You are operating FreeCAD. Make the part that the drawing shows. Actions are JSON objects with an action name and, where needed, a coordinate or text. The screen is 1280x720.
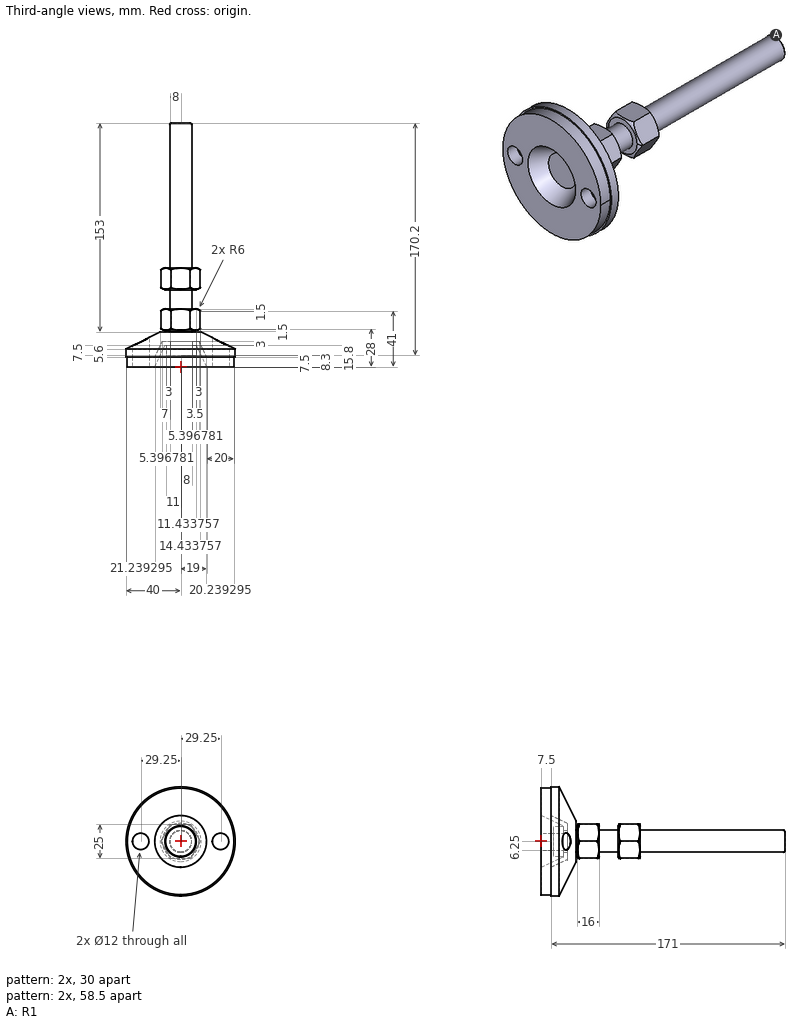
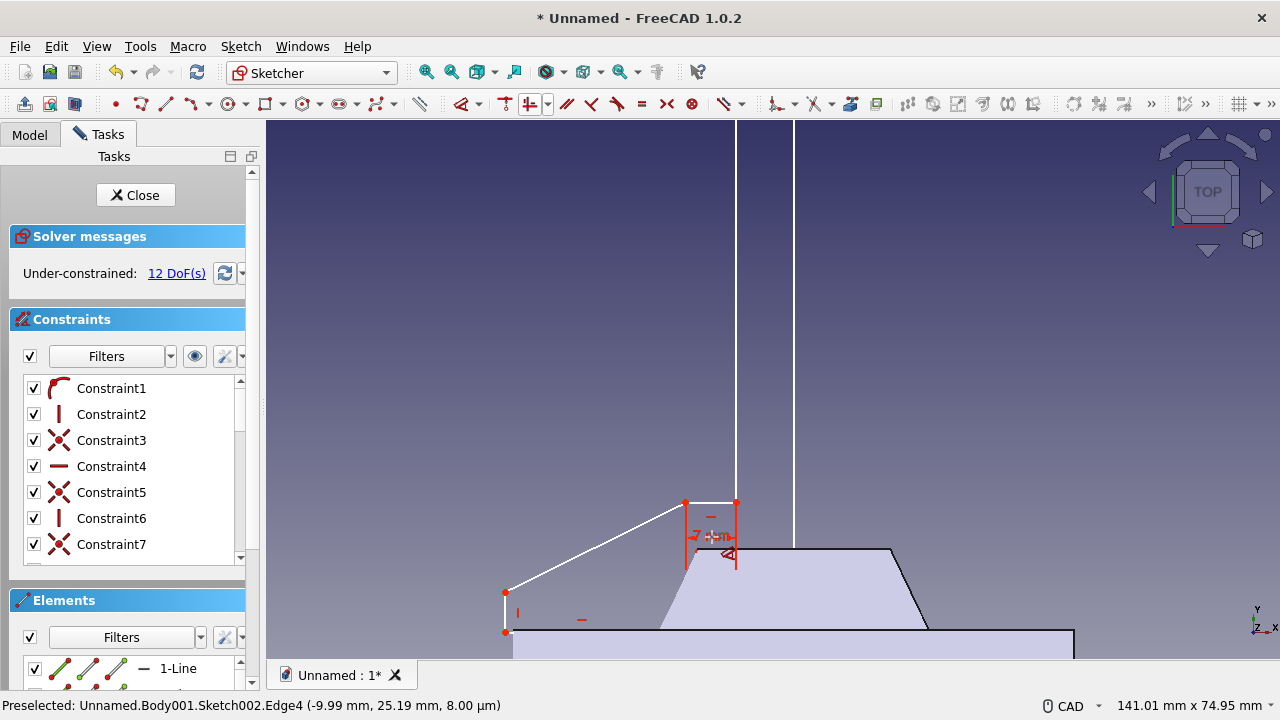
{"action": "scroll", "coordinate": [736, 561], "scroll_direction": "up", "scroll_amount": 4}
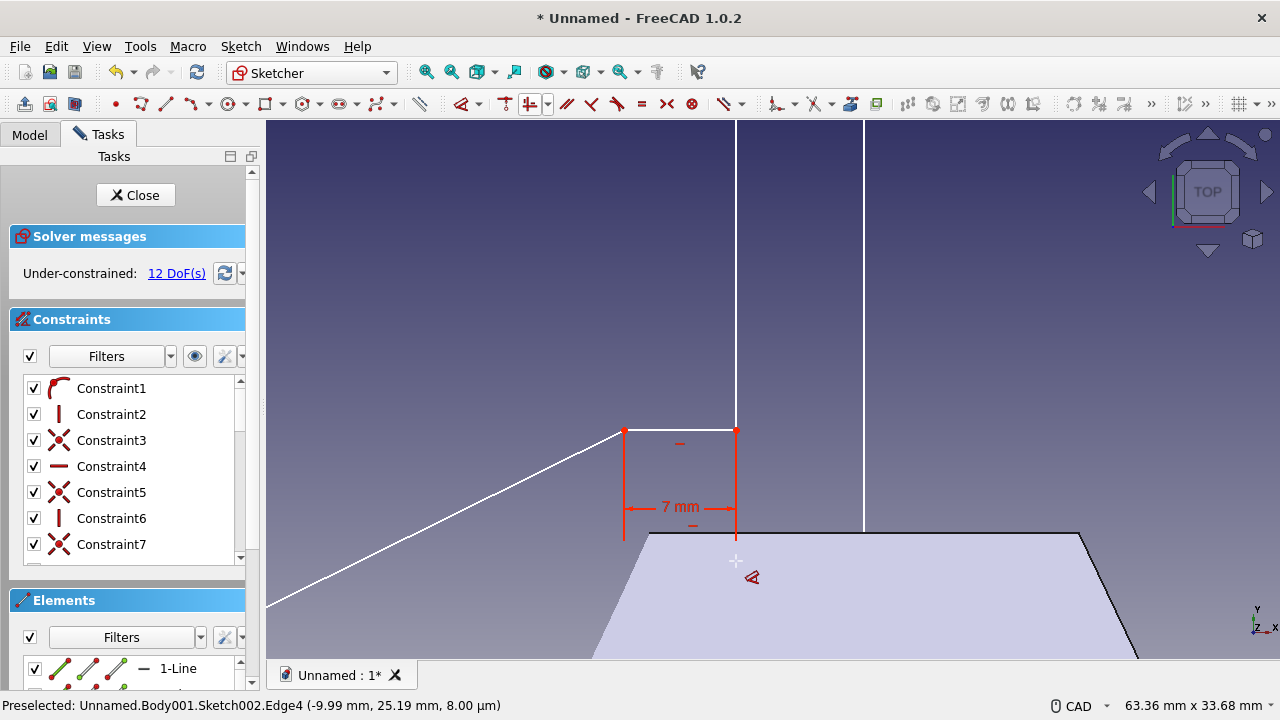
{"action": "left_click", "coordinate": [736, 561]}
{"action": "left_click", "coordinate": [770, 561]}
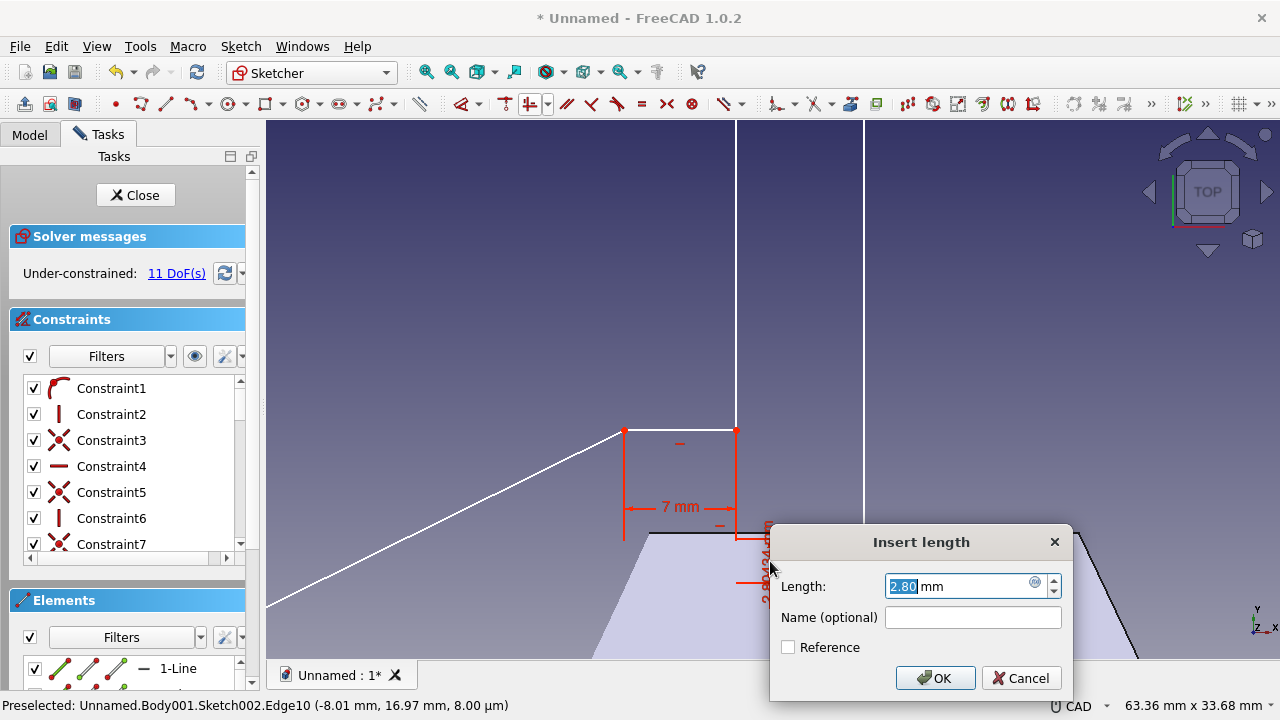
{"action": "type", "text": "3"}
{"action": "key", "text": "Return"}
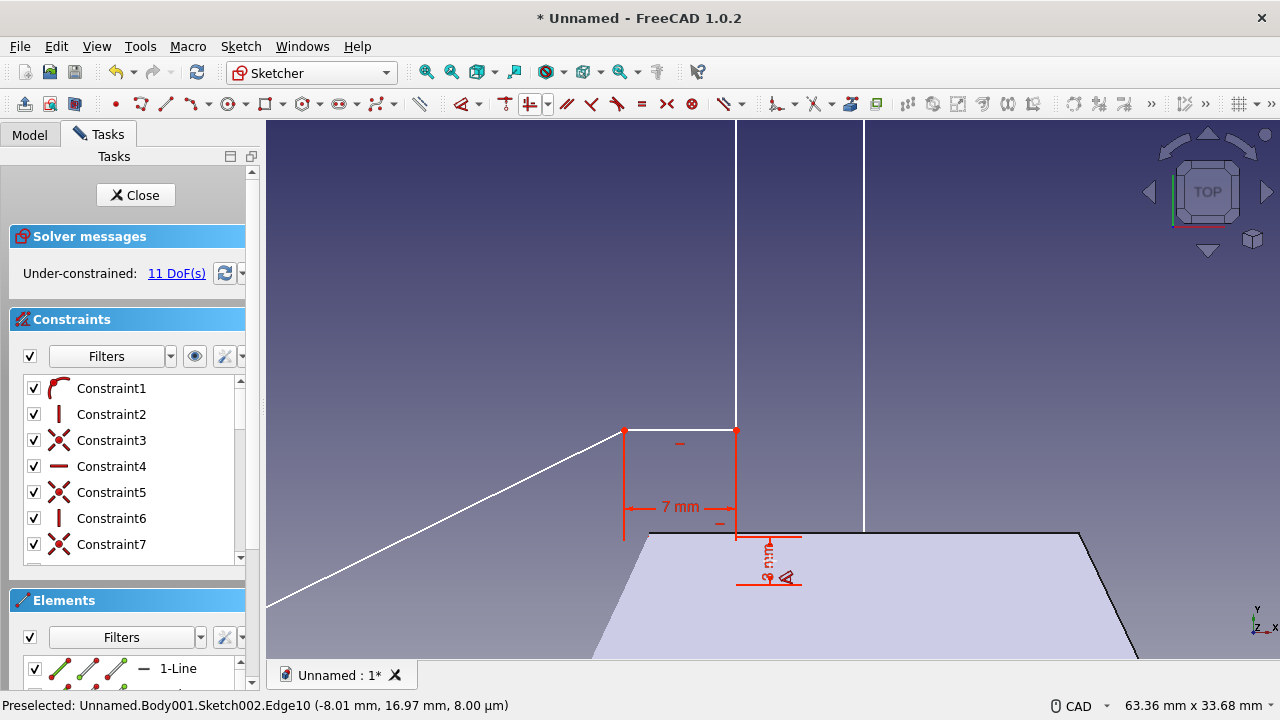
{"action": "left_click", "coordinate": [722, 585]}
{"action": "left_click", "coordinate": [712, 619]}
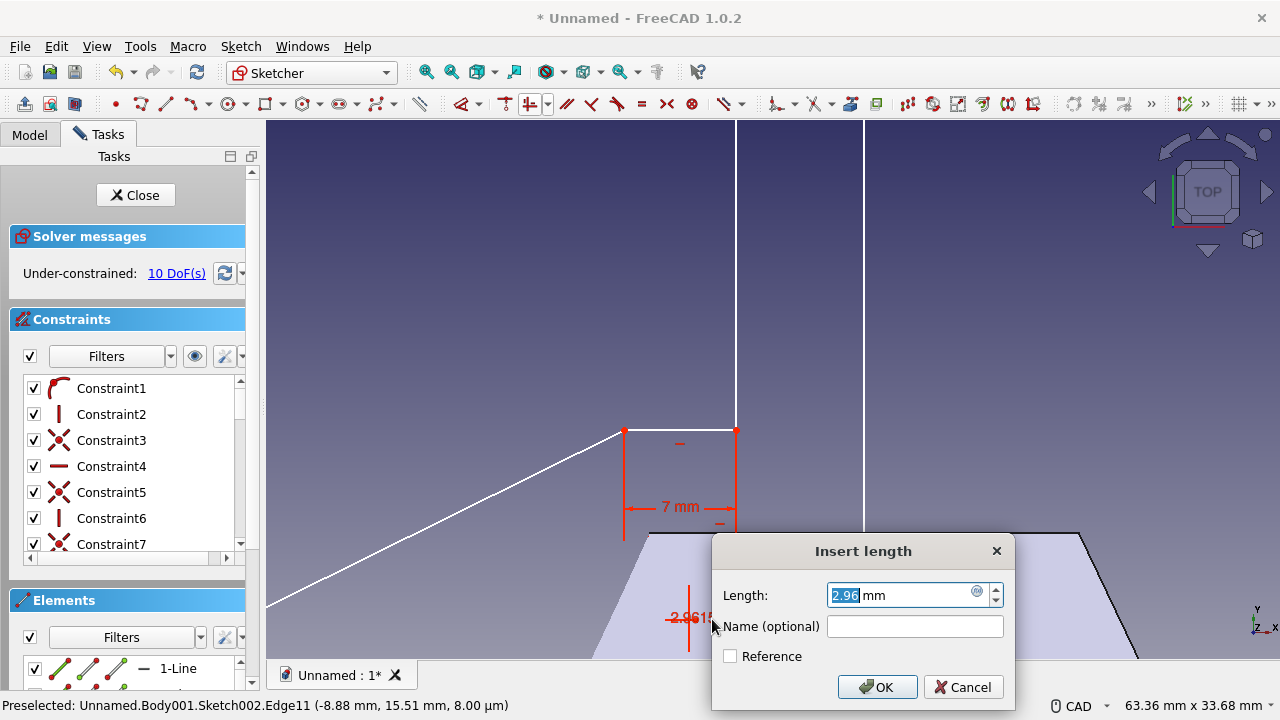
{"action": "type", "text": "3"}
{"action": "key", "text": "Return"}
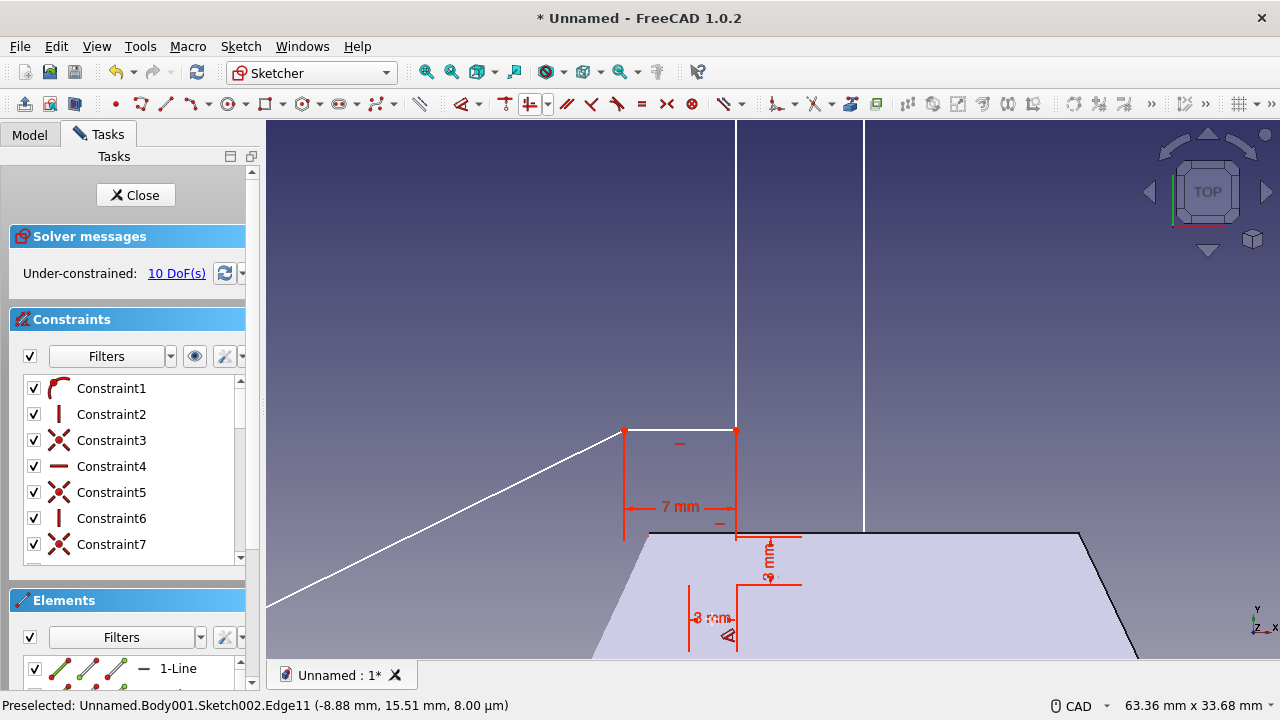
{"action": "scroll", "coordinate": [724, 512], "scroll_direction": "down", "scroll_amount": 11}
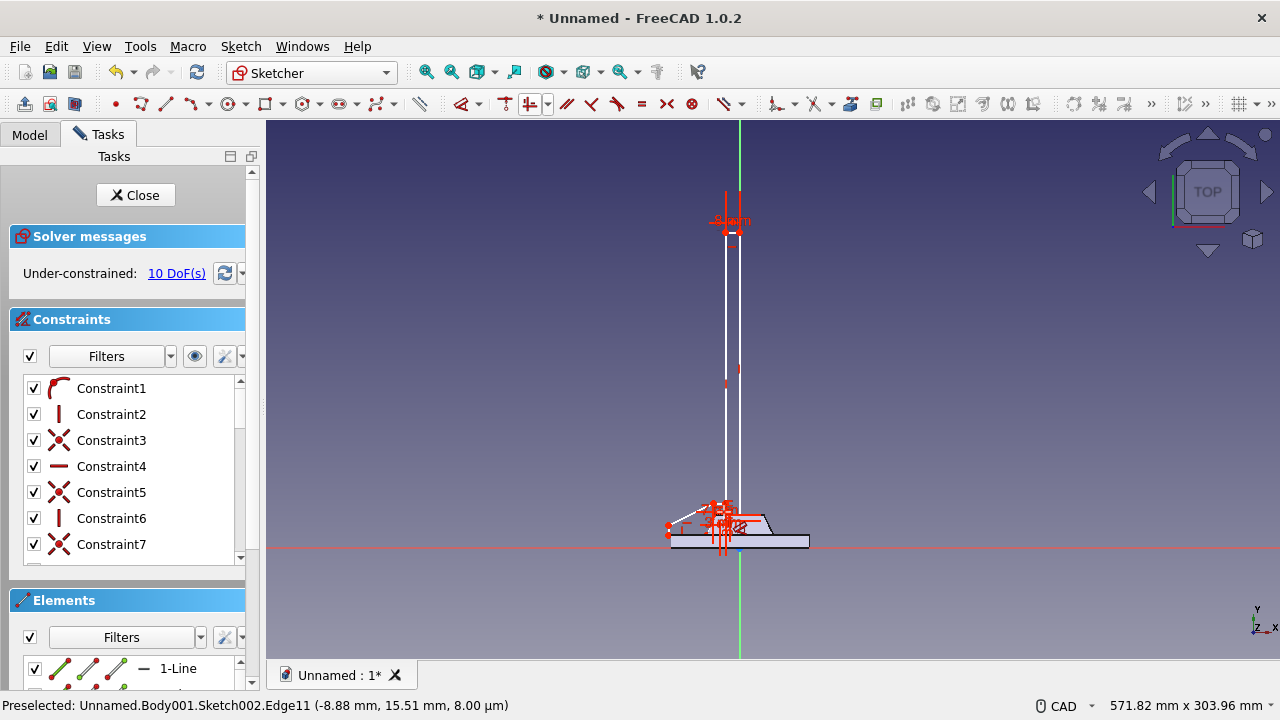
{"action": "scroll", "coordinate": [726, 535], "scroll_direction": "up", "scroll_amount": 5}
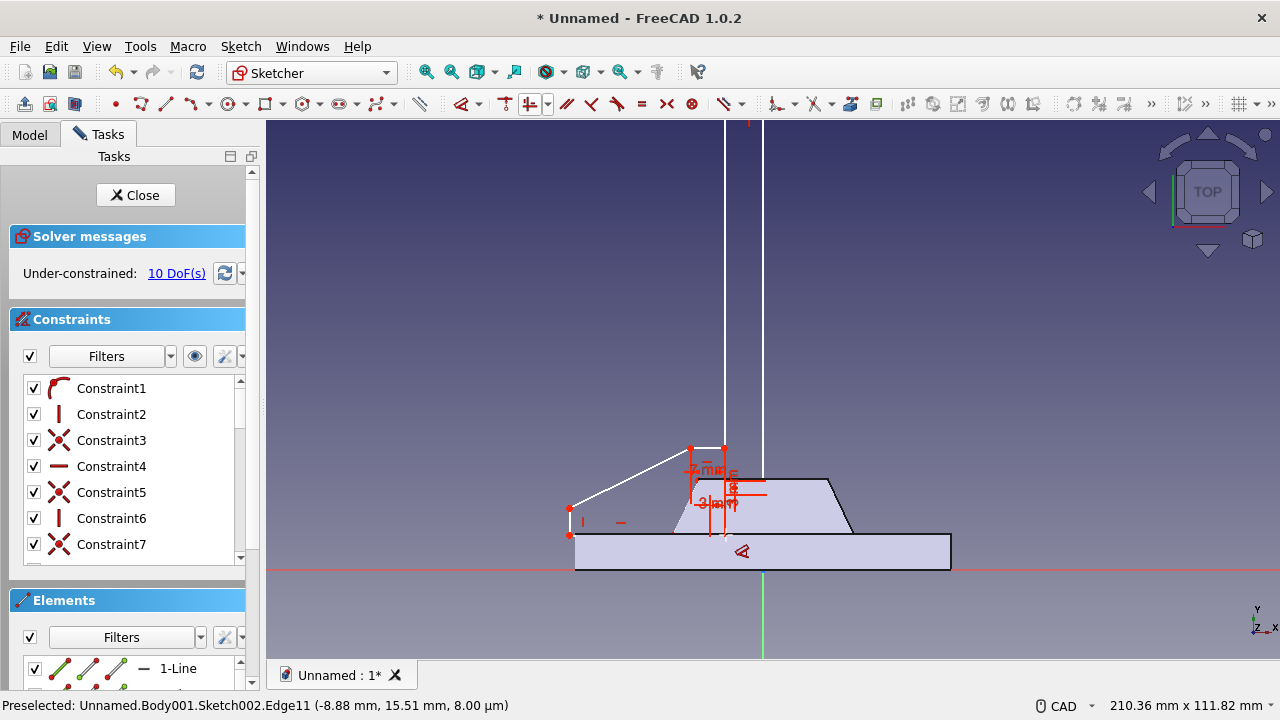
{"action": "left_click", "coordinate": [726, 533]}
{"action": "left_click", "coordinate": [737, 591]}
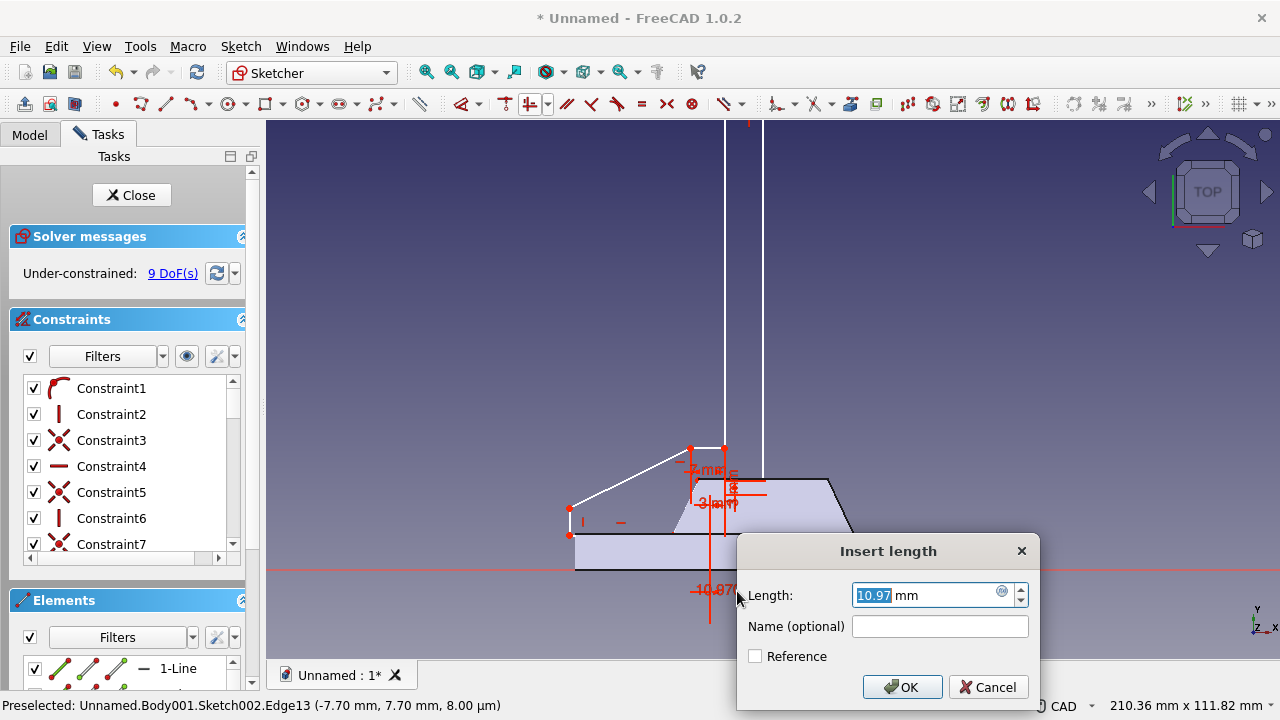
{"action": "type", "text": "11"}
{"action": "key", "text": "Return"}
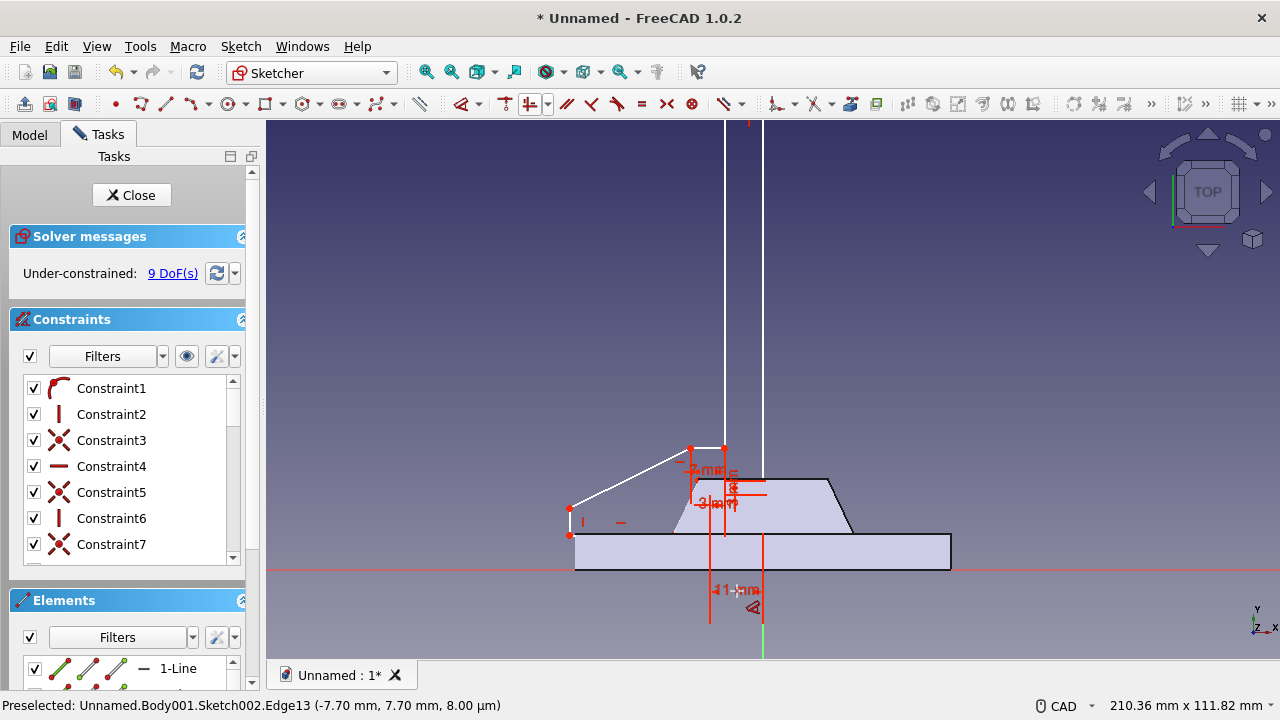
{"action": "left_click", "coordinate": [725, 227]}
{"action": "left_click", "coordinate": [691, 298]}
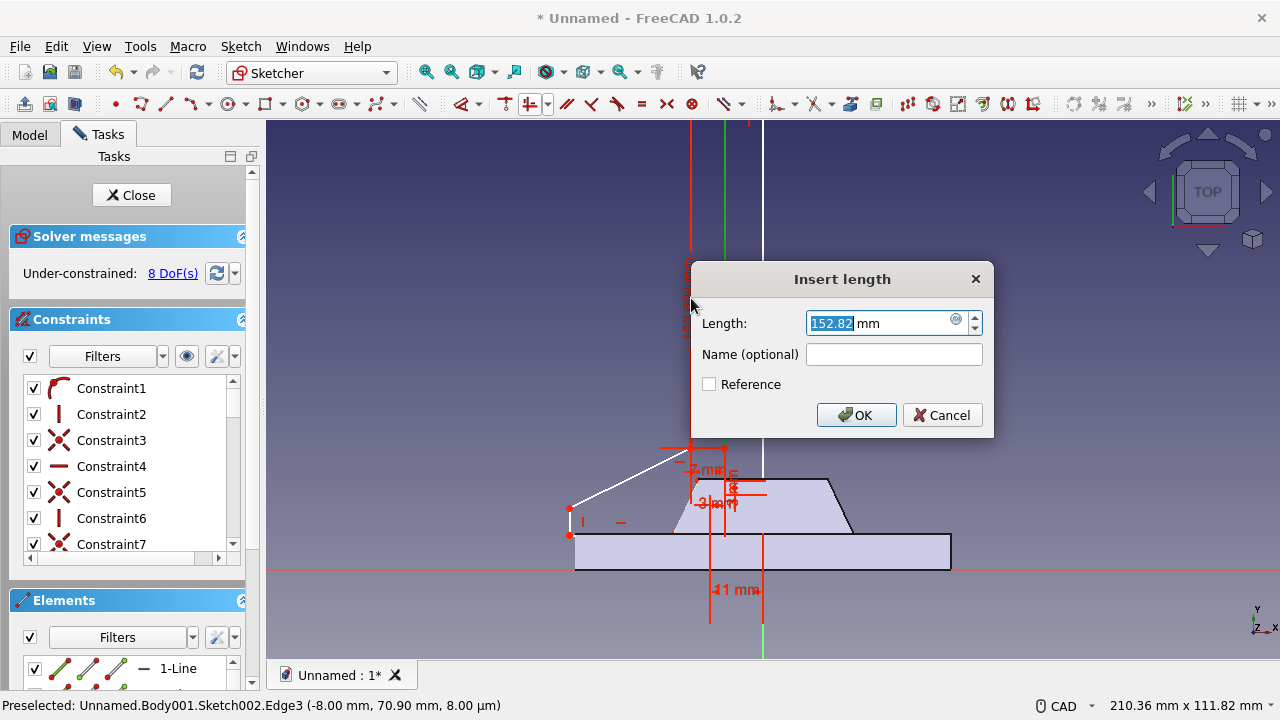
{"action": "type", "text": "153"}
{"action": "key", "text": "Return"}